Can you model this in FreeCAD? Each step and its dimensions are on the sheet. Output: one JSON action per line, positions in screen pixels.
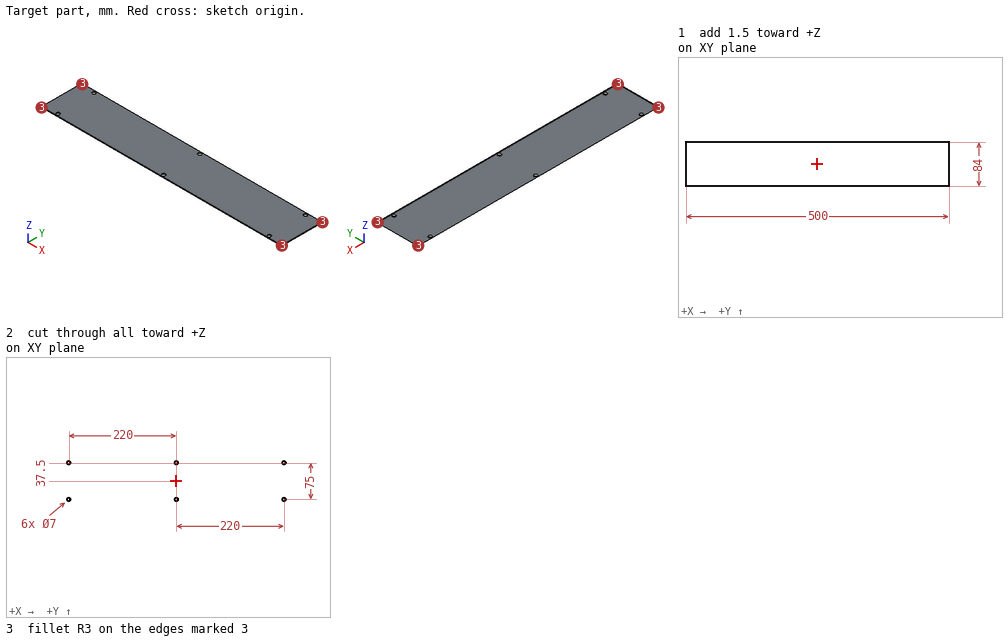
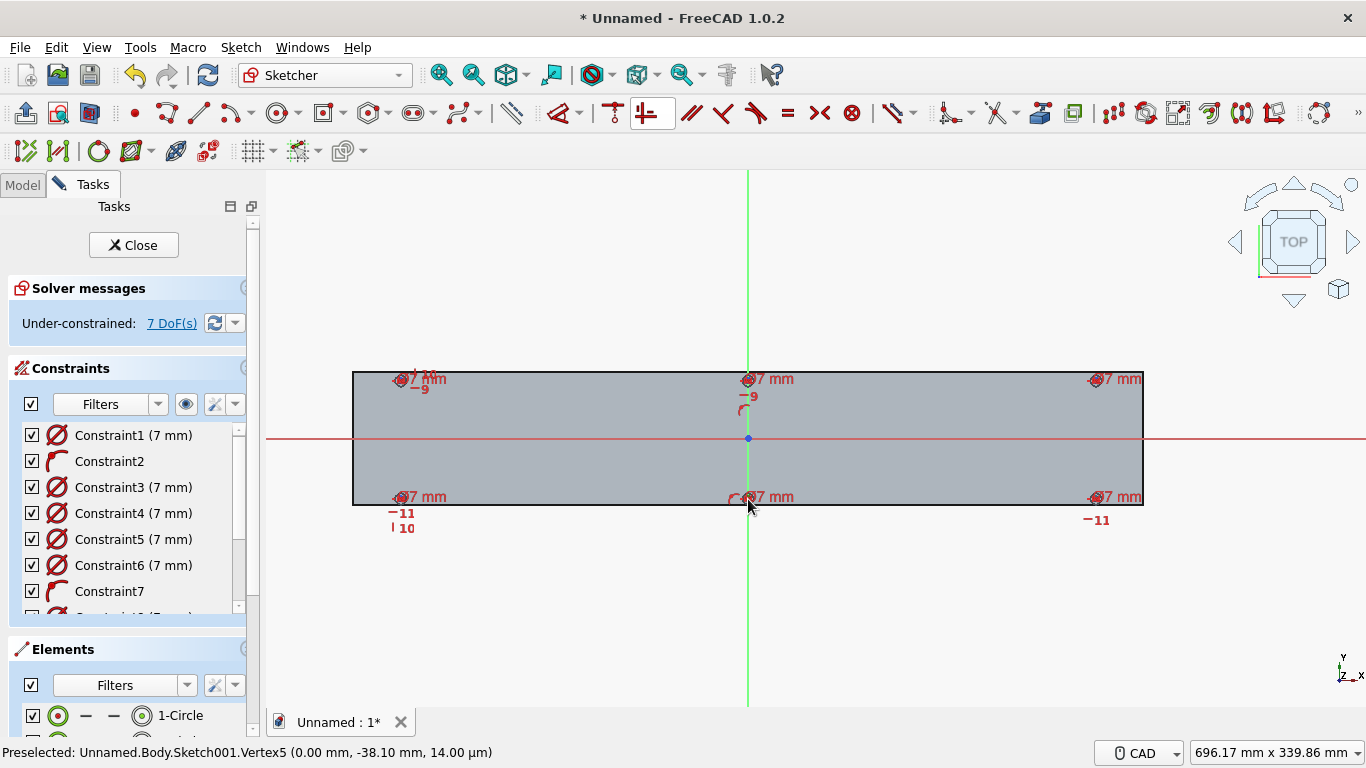
{"action": "key", "text": "h"}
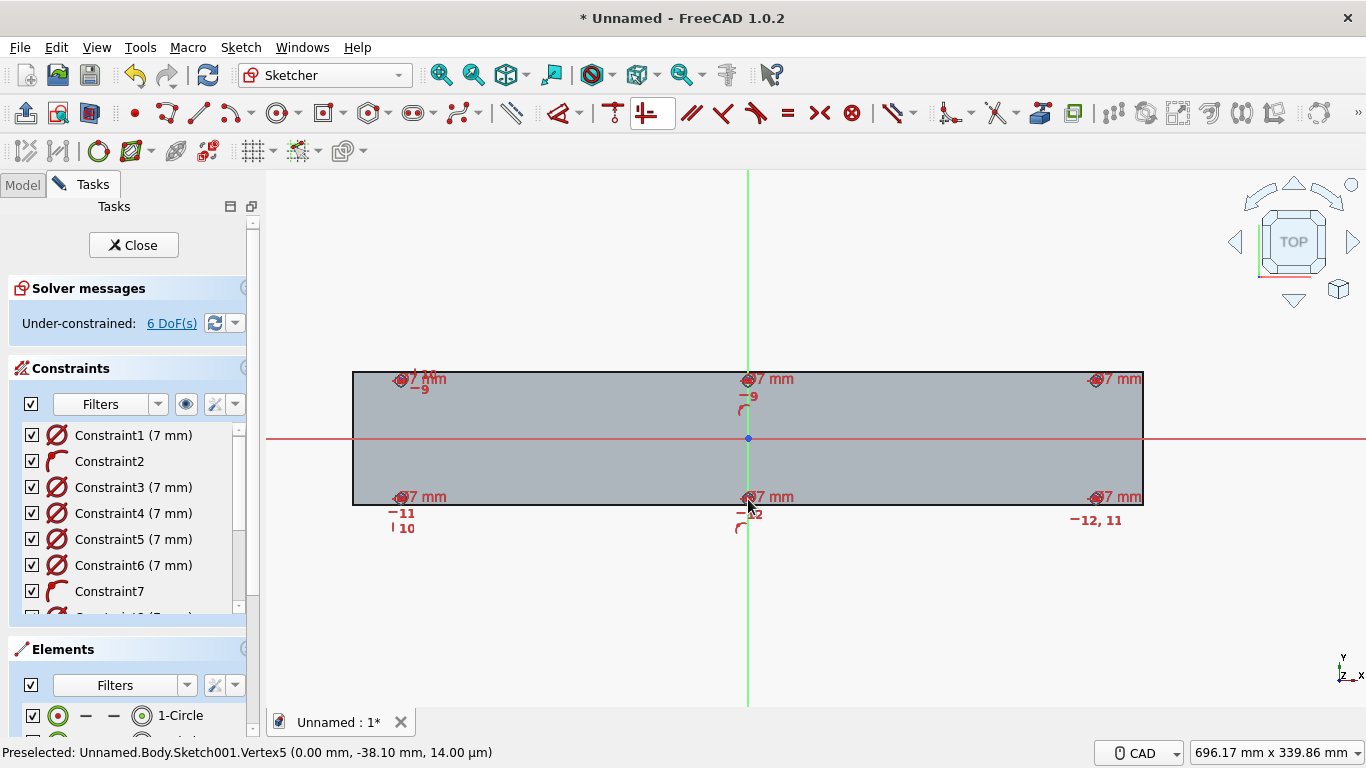
{"action": "left_click", "coordinate": [1096, 499]}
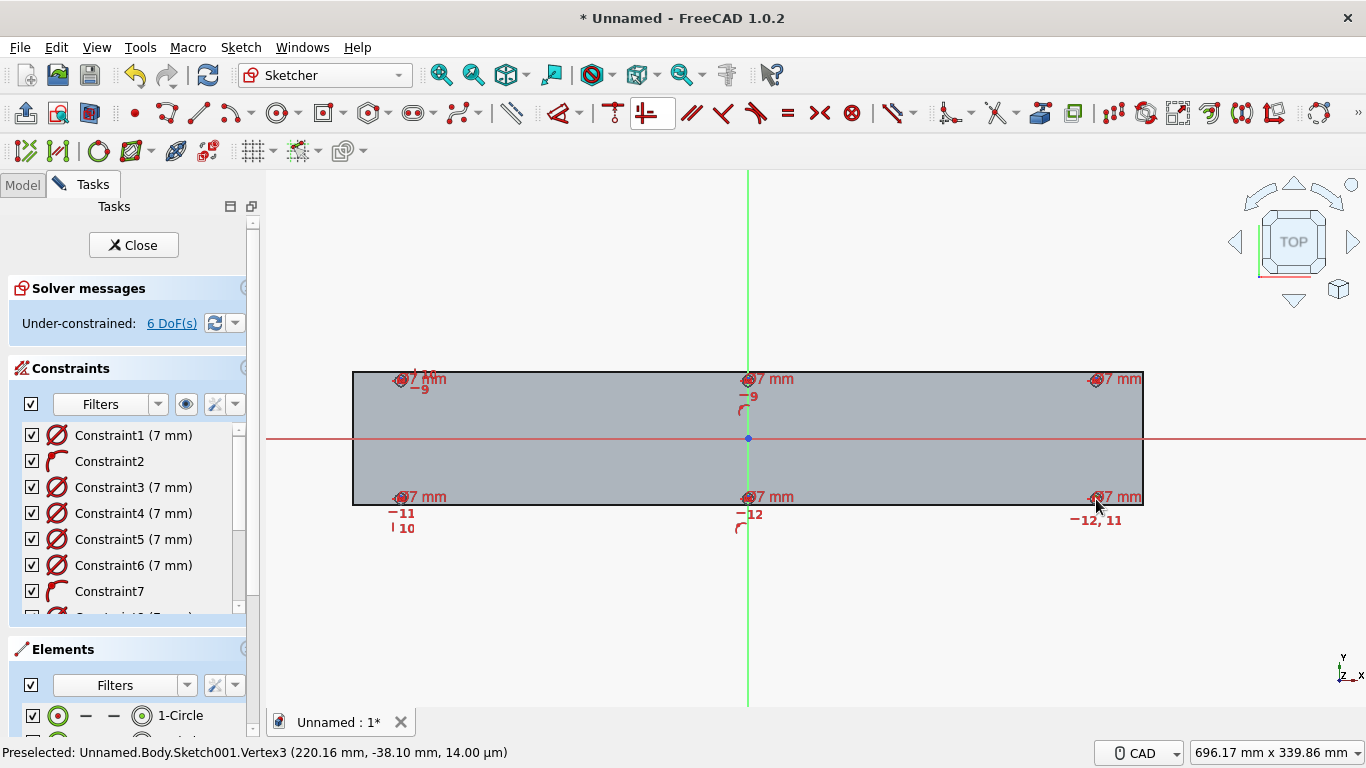
{"action": "left_click", "coordinate": [1096, 381]}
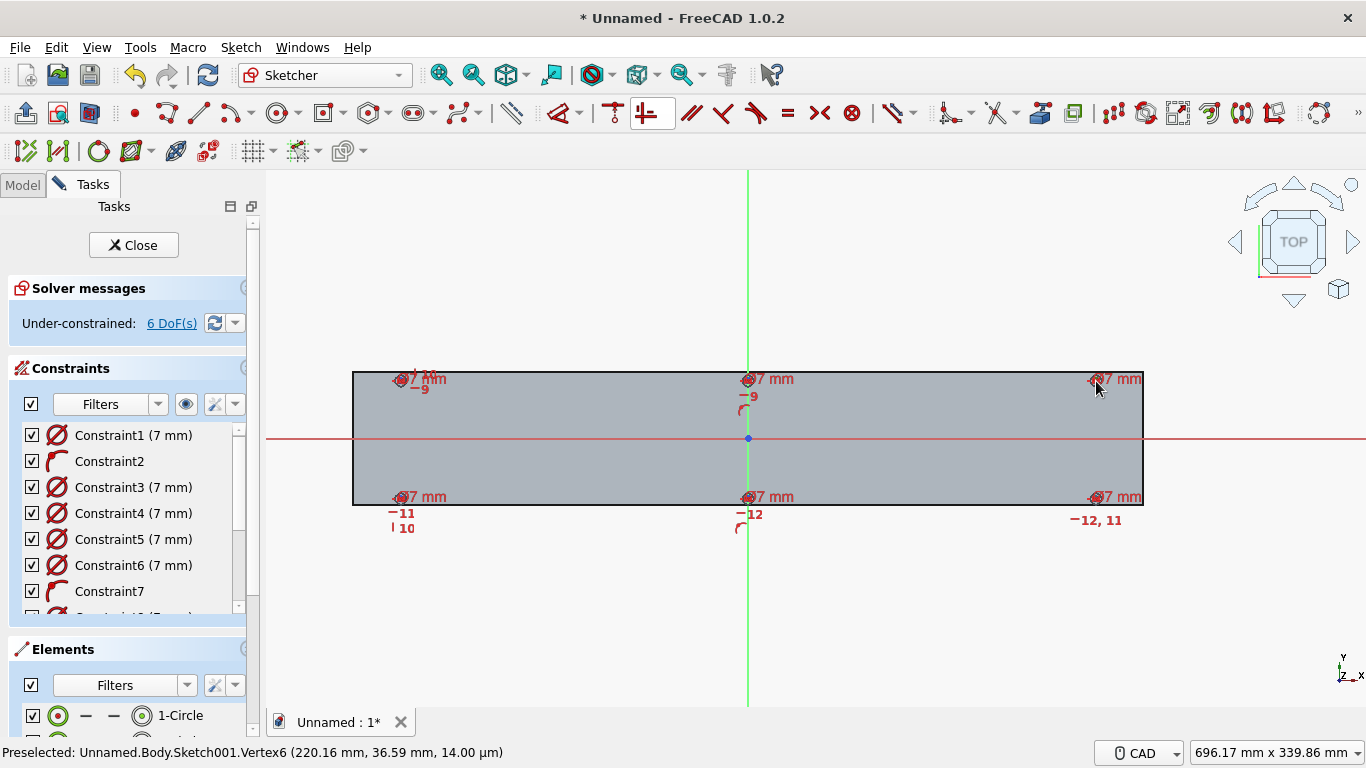
{"action": "key", "text": "v"}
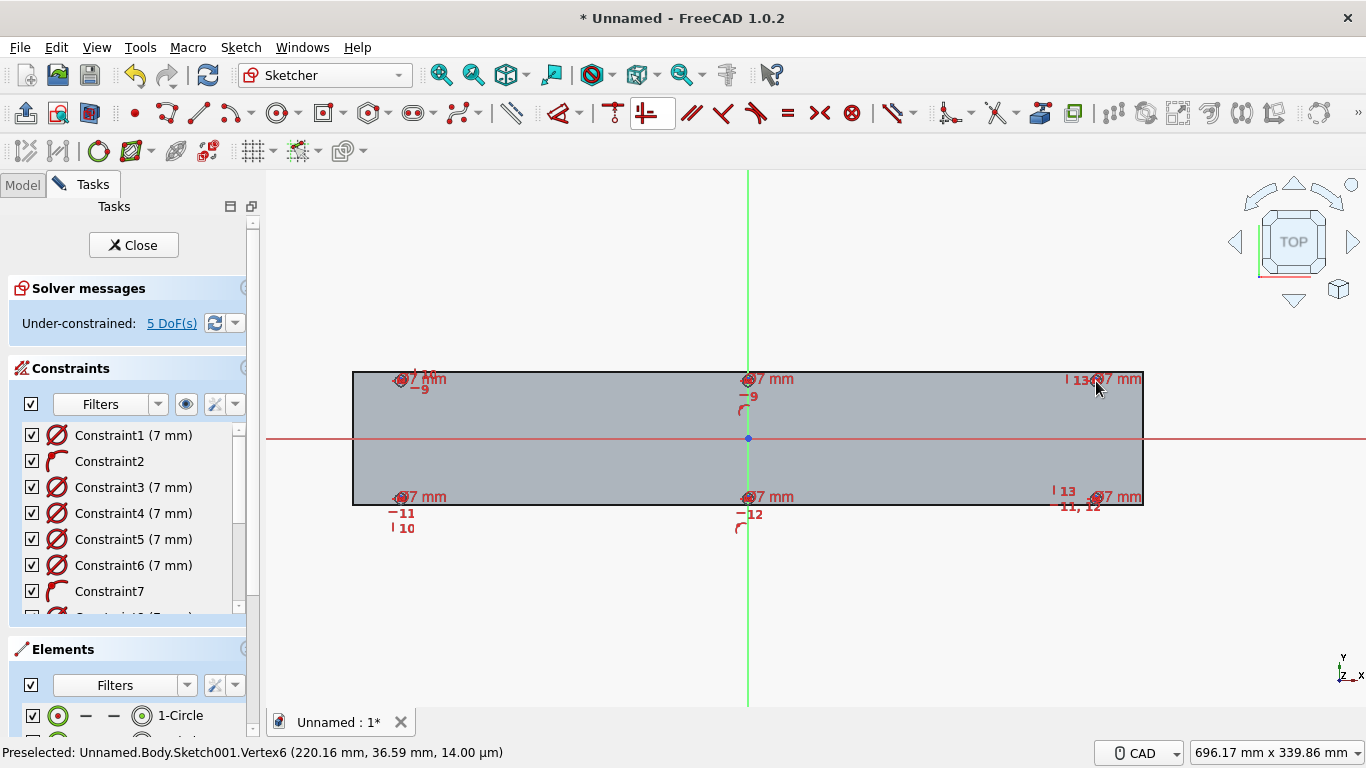
{"action": "left_click", "coordinate": [748, 381]}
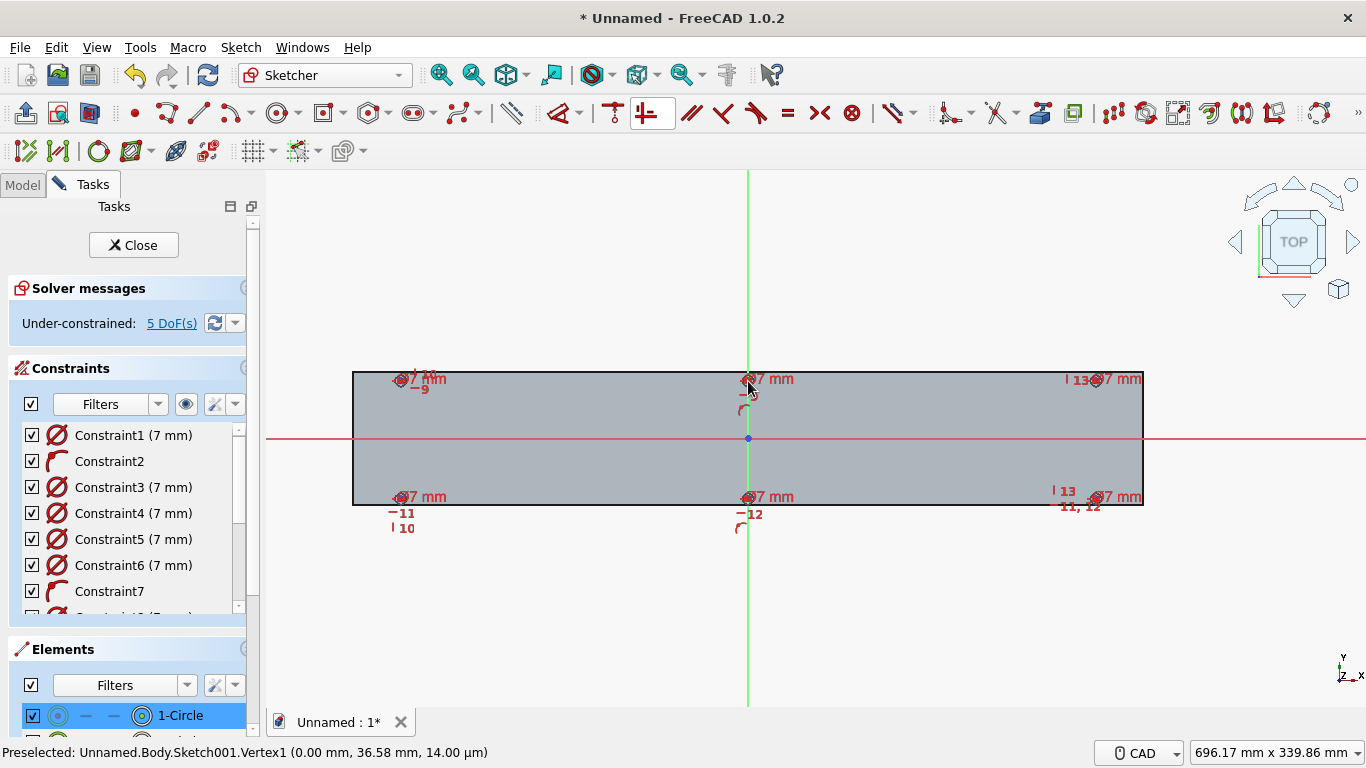
{"action": "left_click", "coordinate": [1096, 381]}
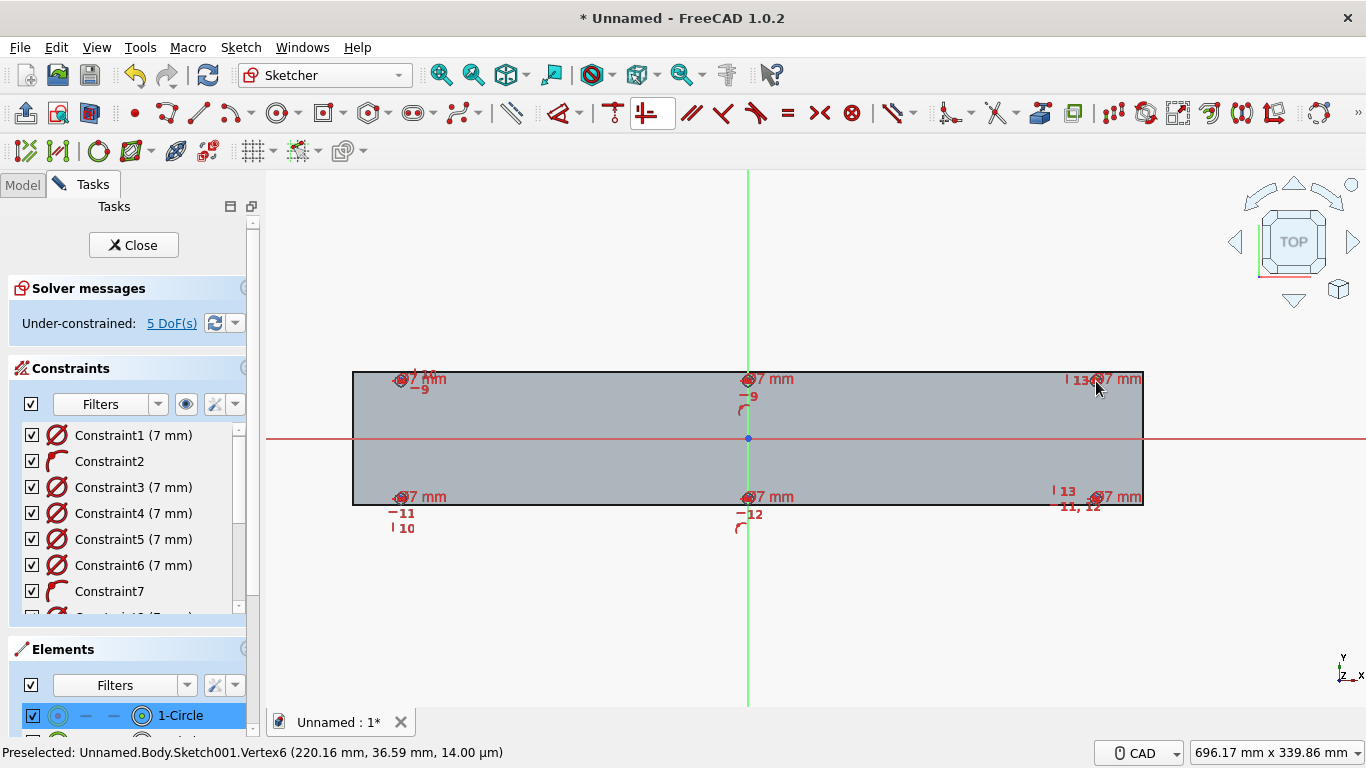
{"action": "left_click", "coordinate": [670, 114]}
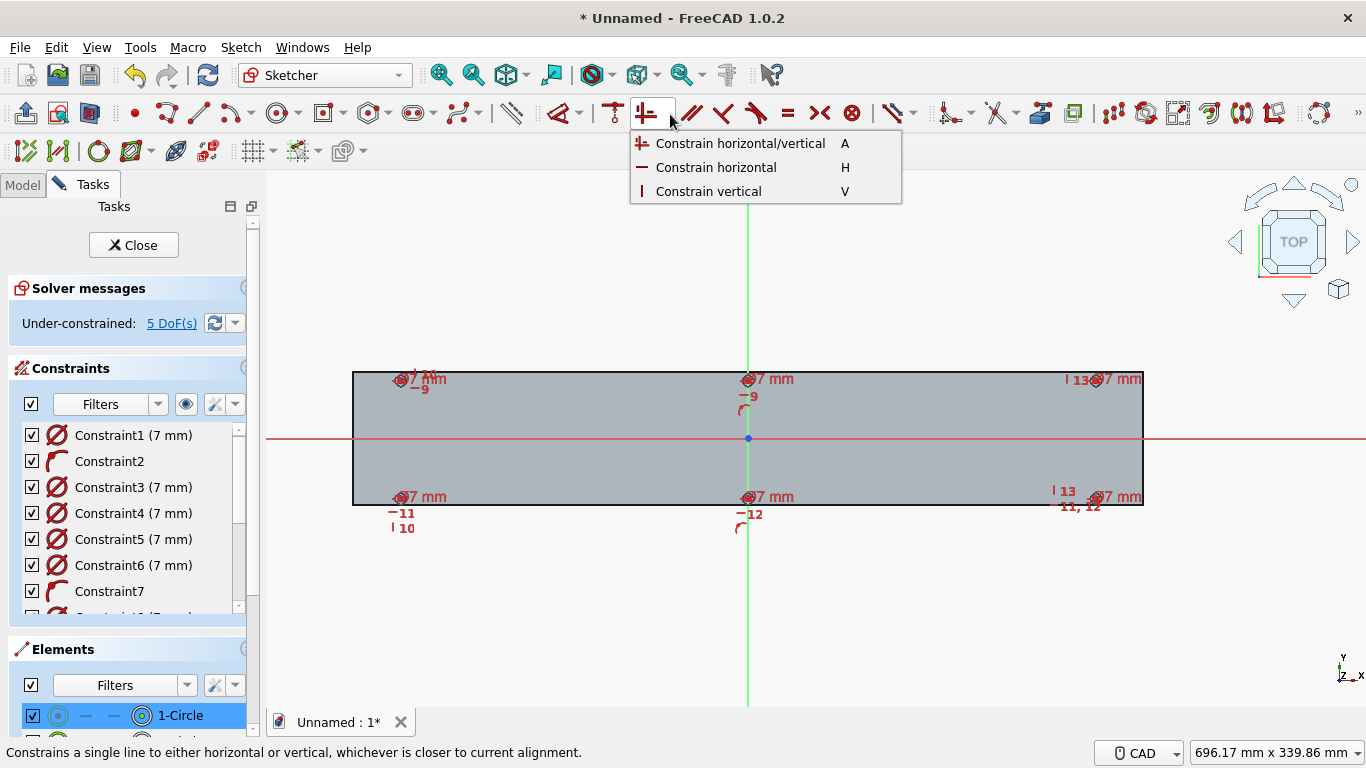
{"action": "left_click", "coordinate": [766, 167]}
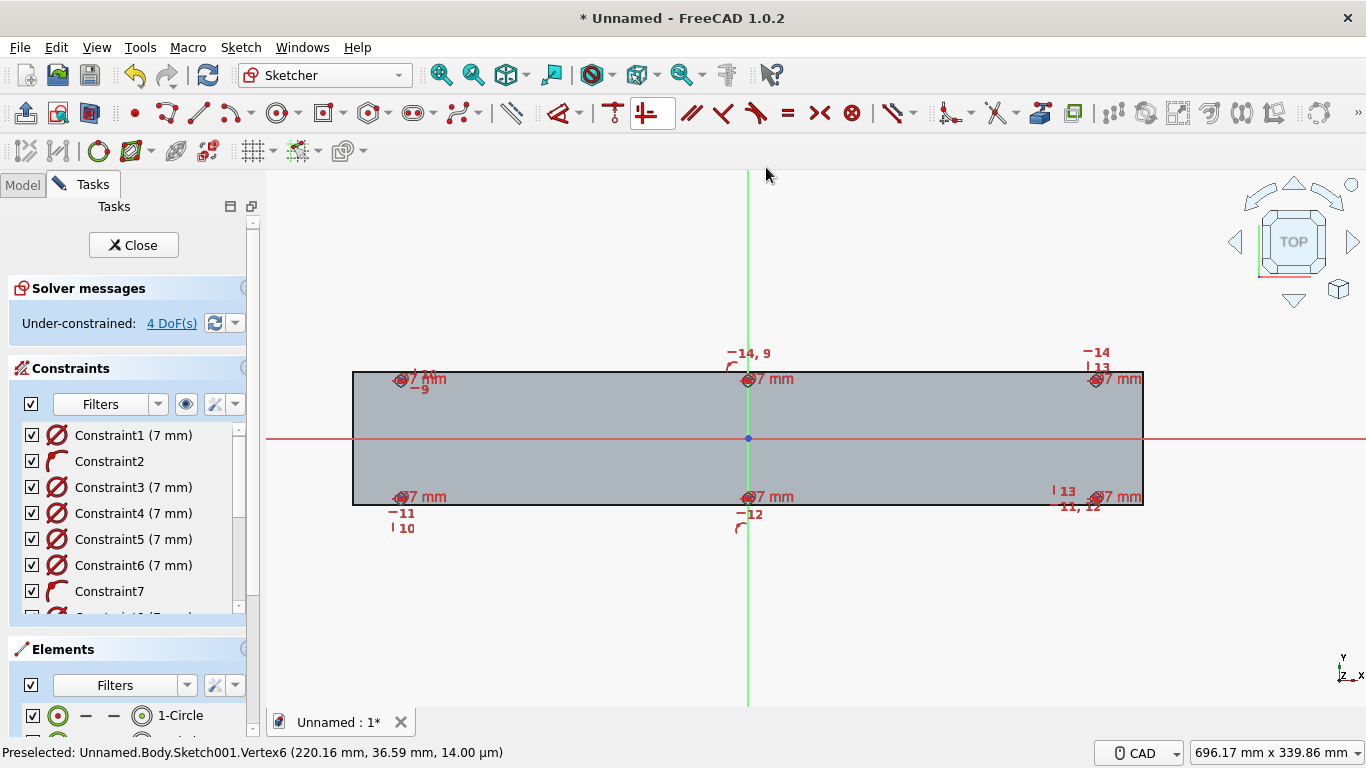
{"action": "left_click", "coordinate": [558, 114]}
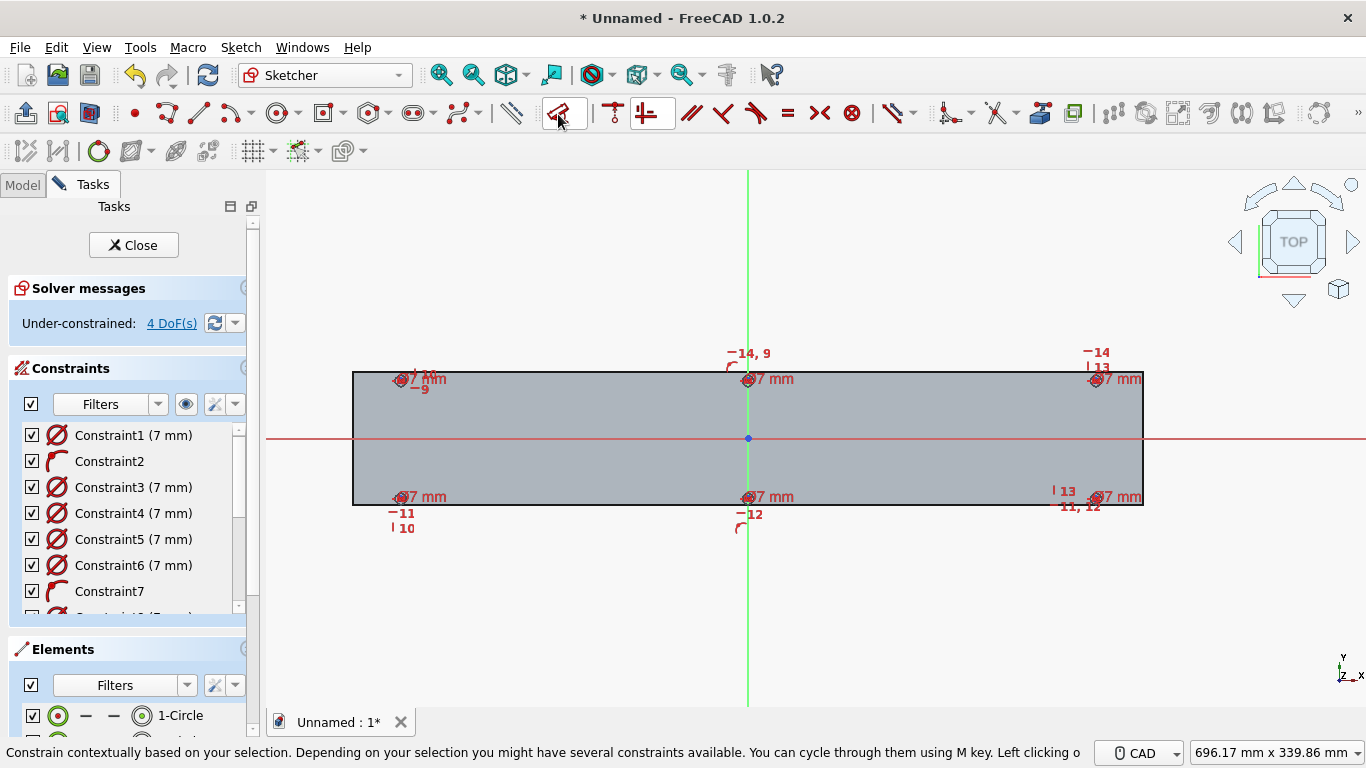
{"action": "left_click", "coordinate": [401, 381]}
{"action": "left_click", "coordinate": [574, 347]}